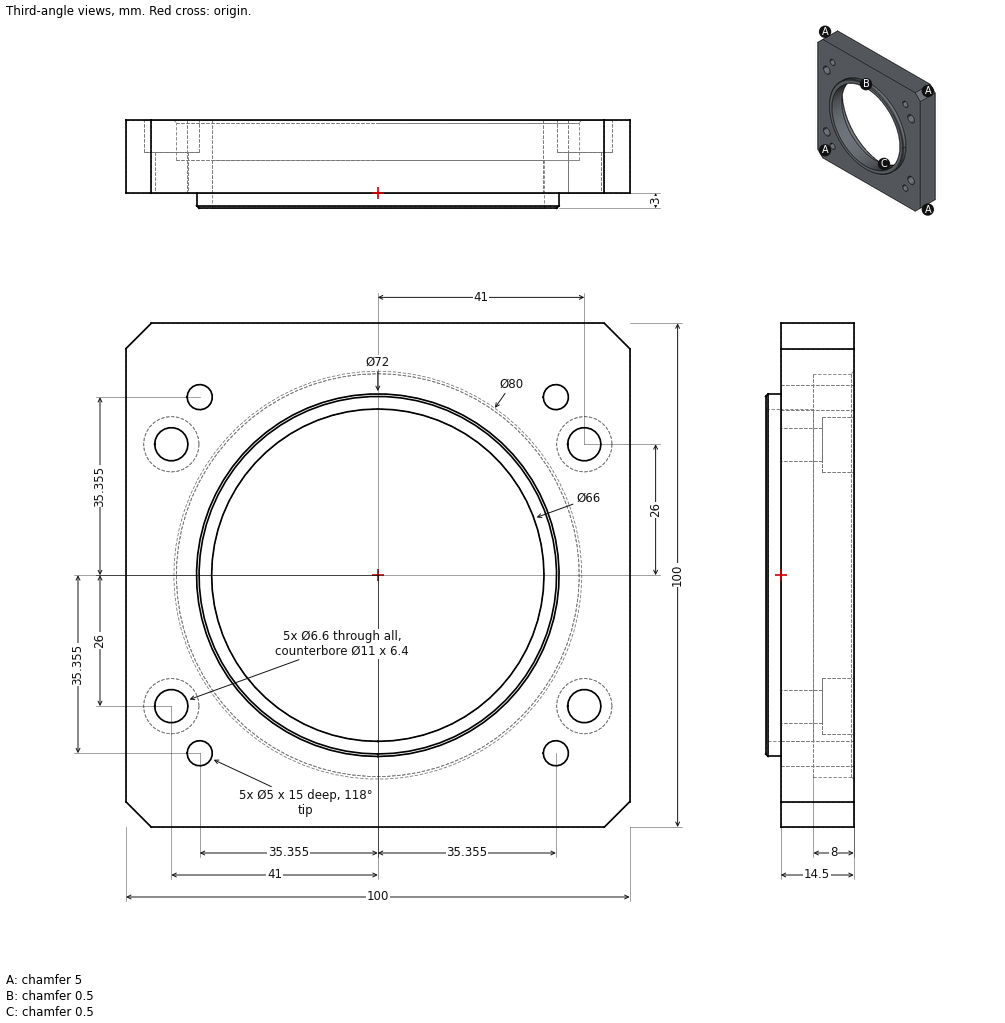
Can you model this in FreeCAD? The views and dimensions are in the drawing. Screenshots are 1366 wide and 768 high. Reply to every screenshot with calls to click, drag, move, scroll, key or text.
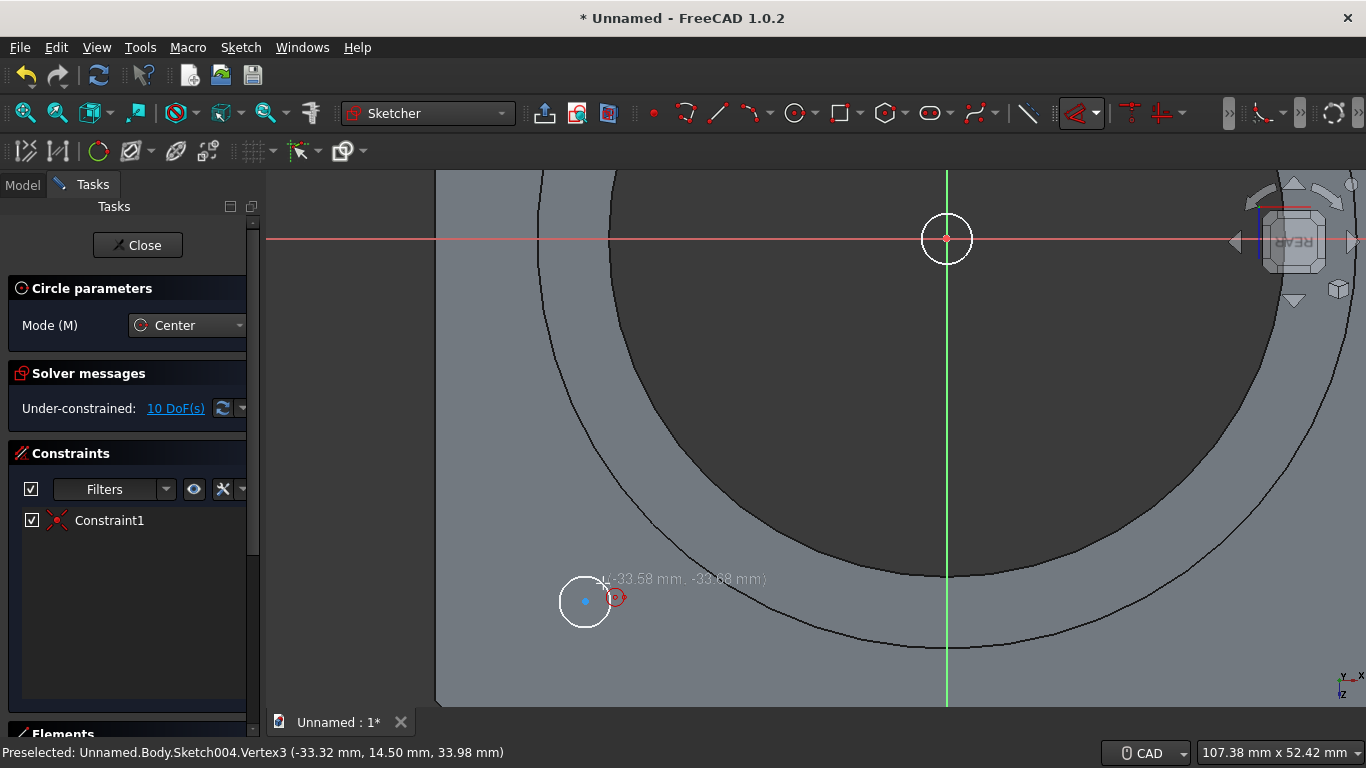
scroll(585, 601, down, 4)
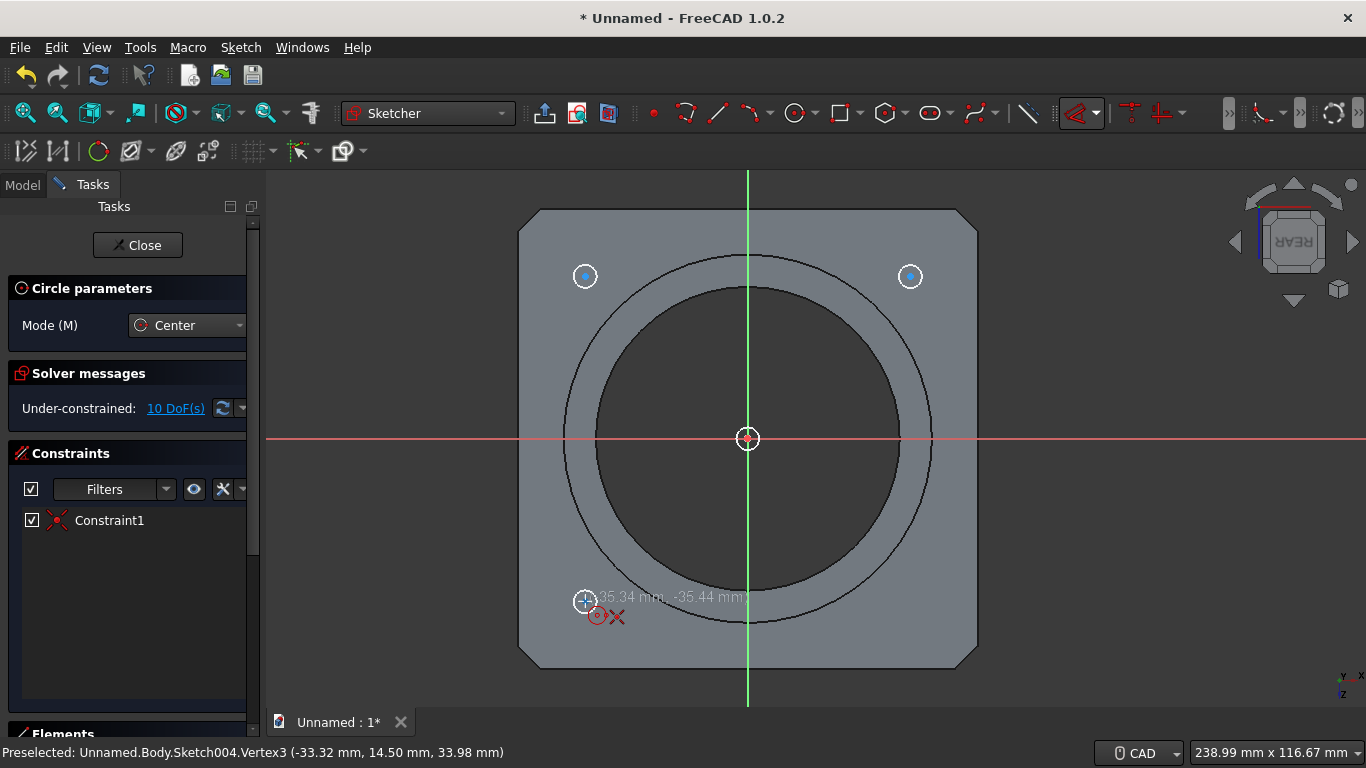
scroll(911, 601, up, 4)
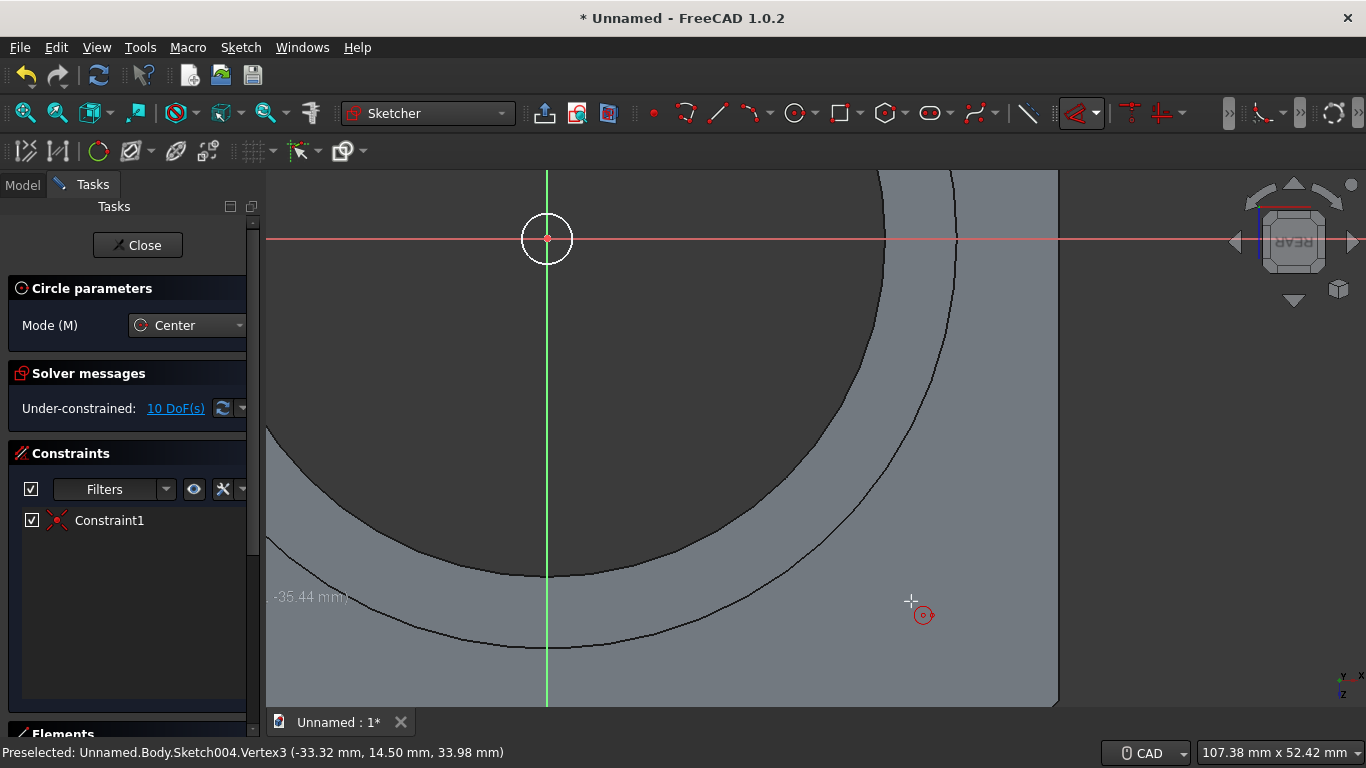
click(909, 601)
click(927, 583)
key(Escape)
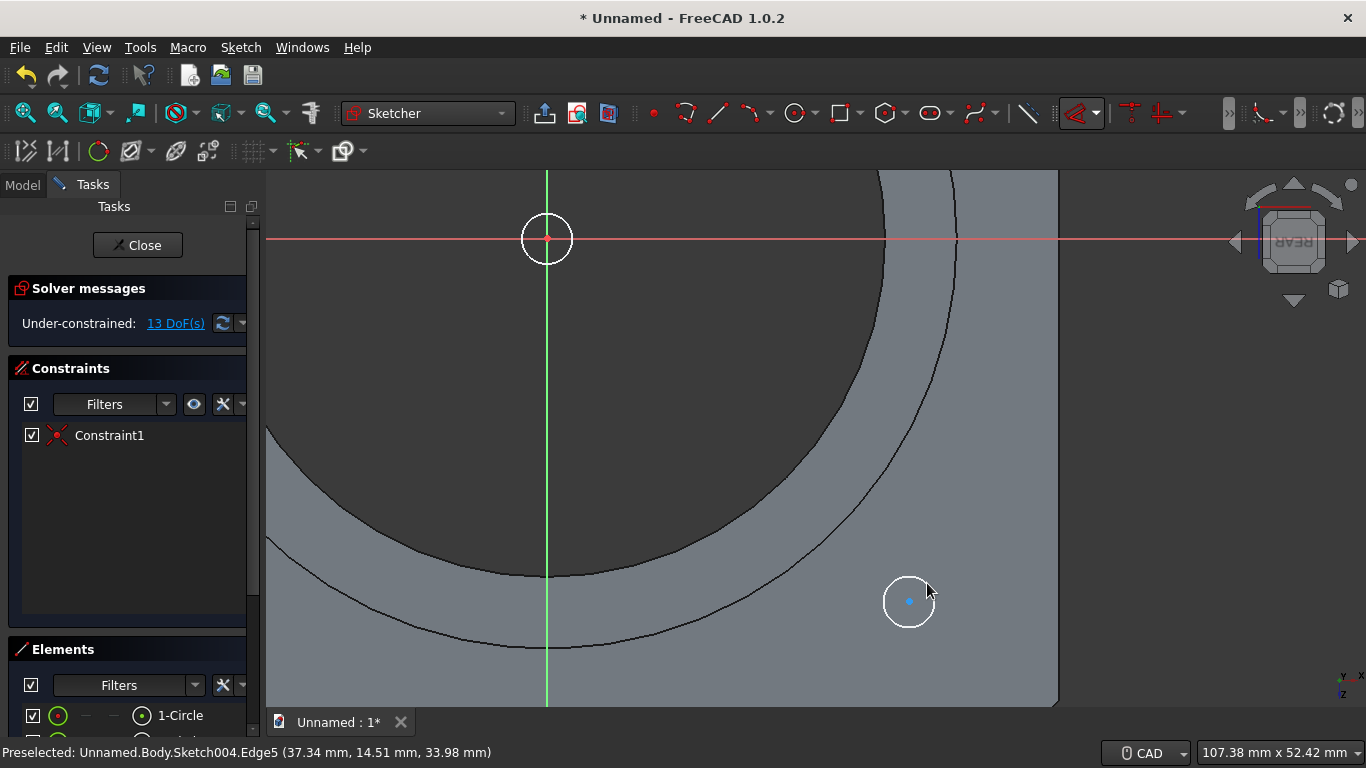
scroll(911, 601, down, 4)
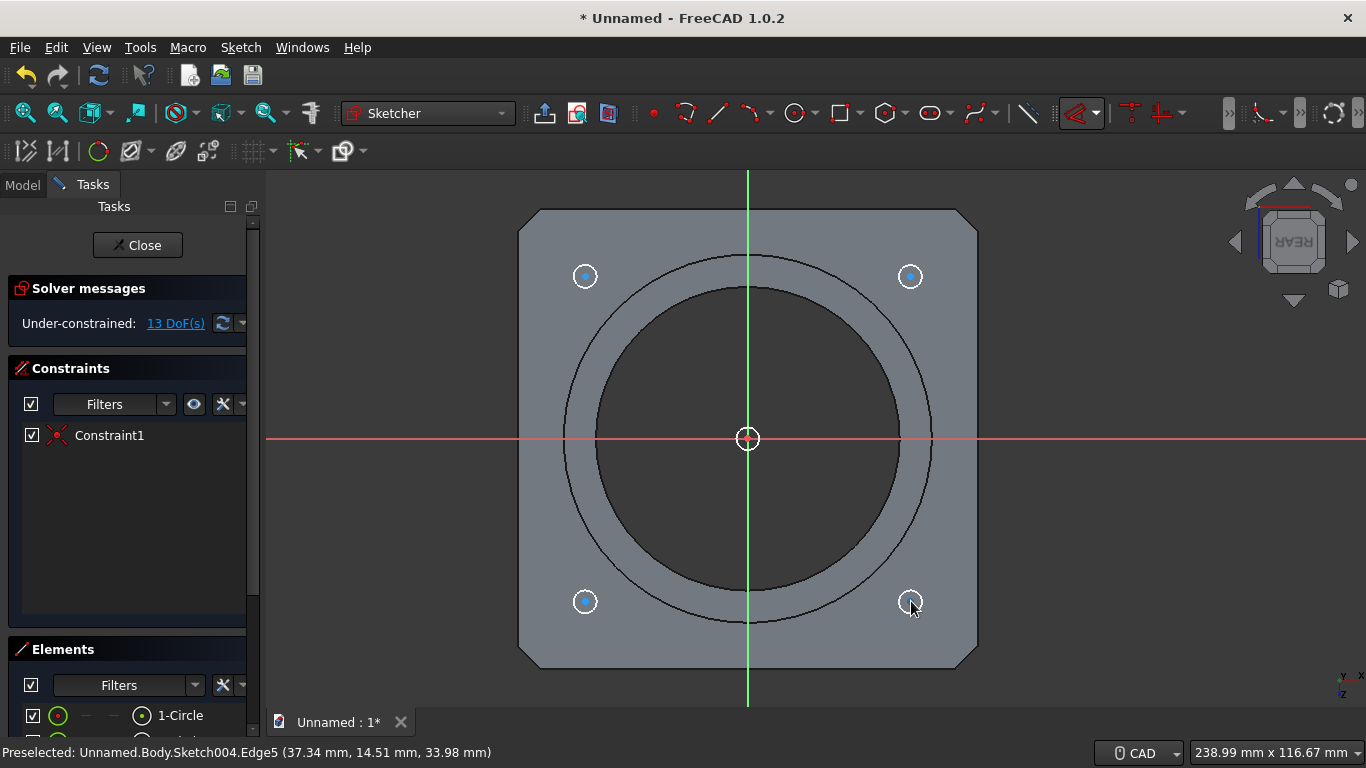
click(593, 268)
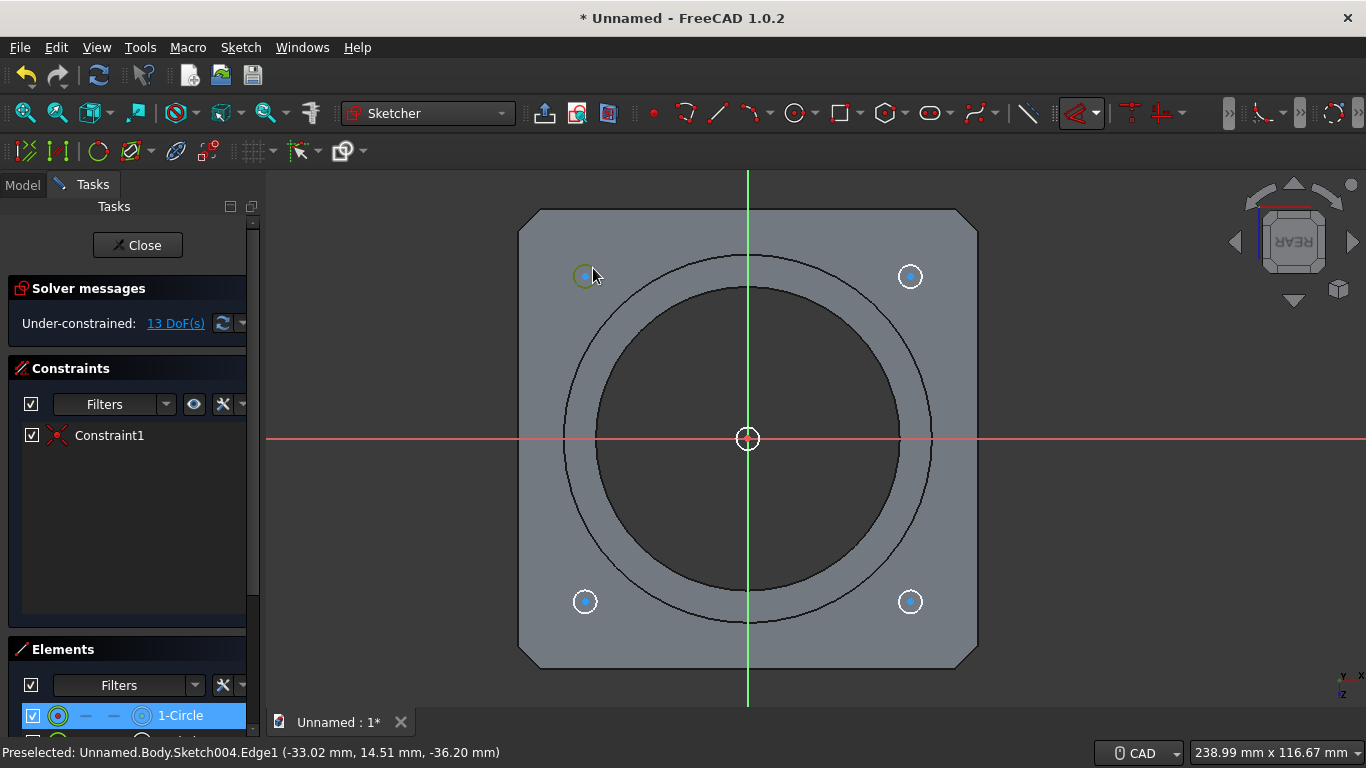
scroll(748, 427, up, 2)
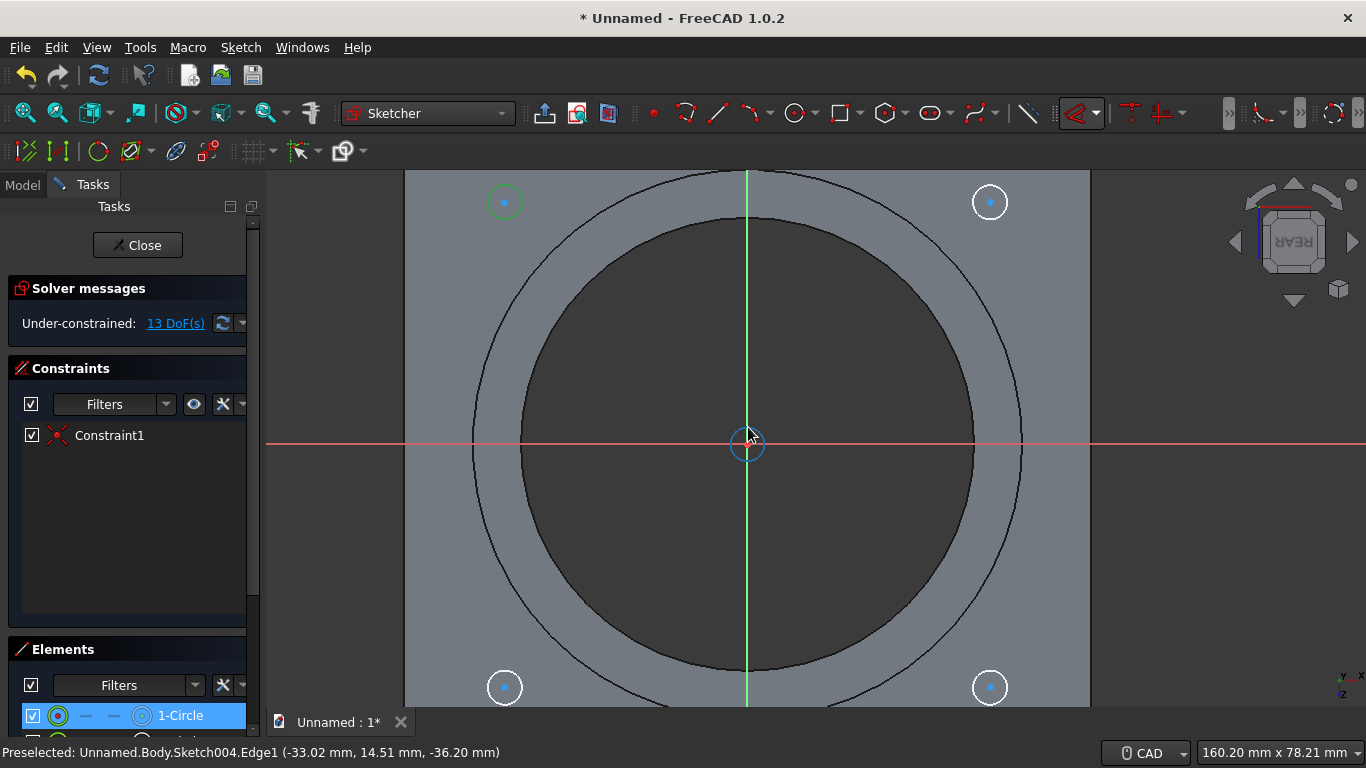
click(748, 427)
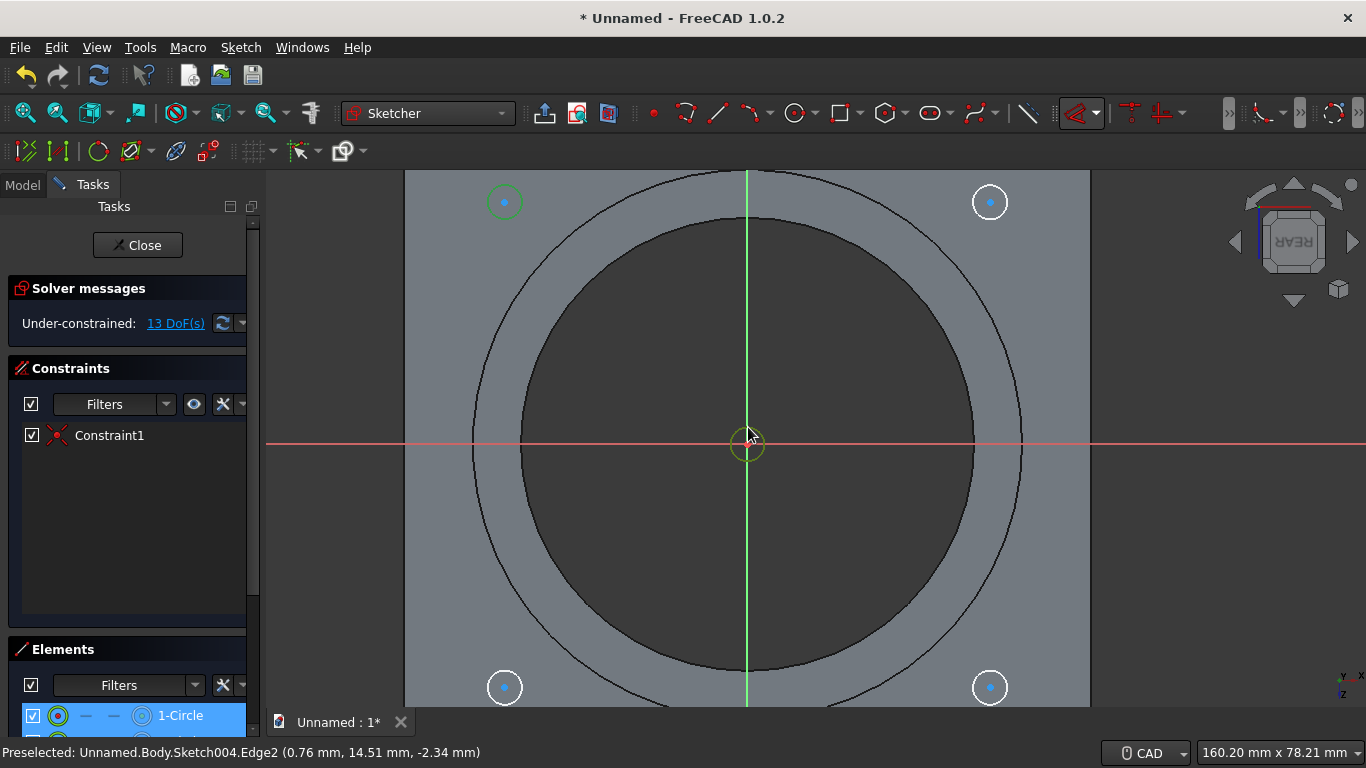
click(978, 214)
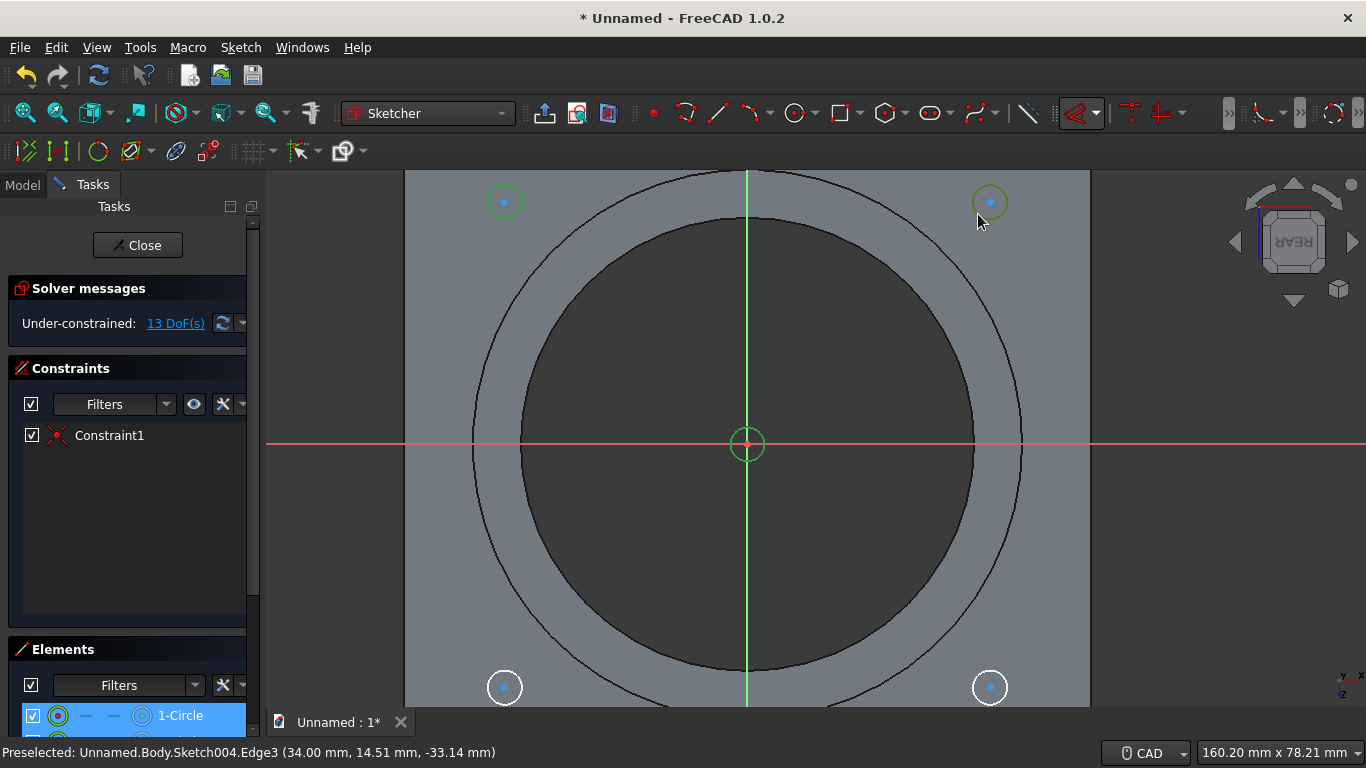
click(517, 676)